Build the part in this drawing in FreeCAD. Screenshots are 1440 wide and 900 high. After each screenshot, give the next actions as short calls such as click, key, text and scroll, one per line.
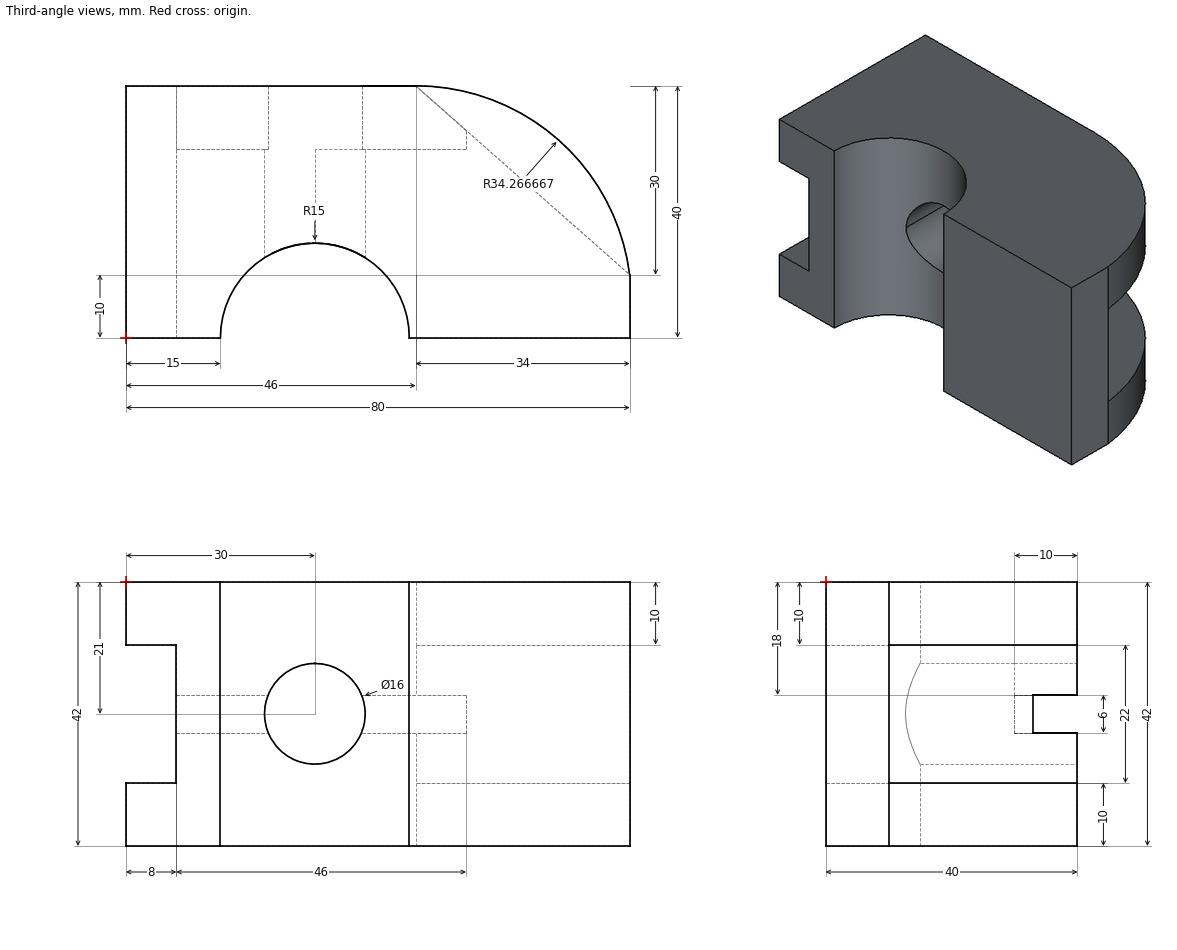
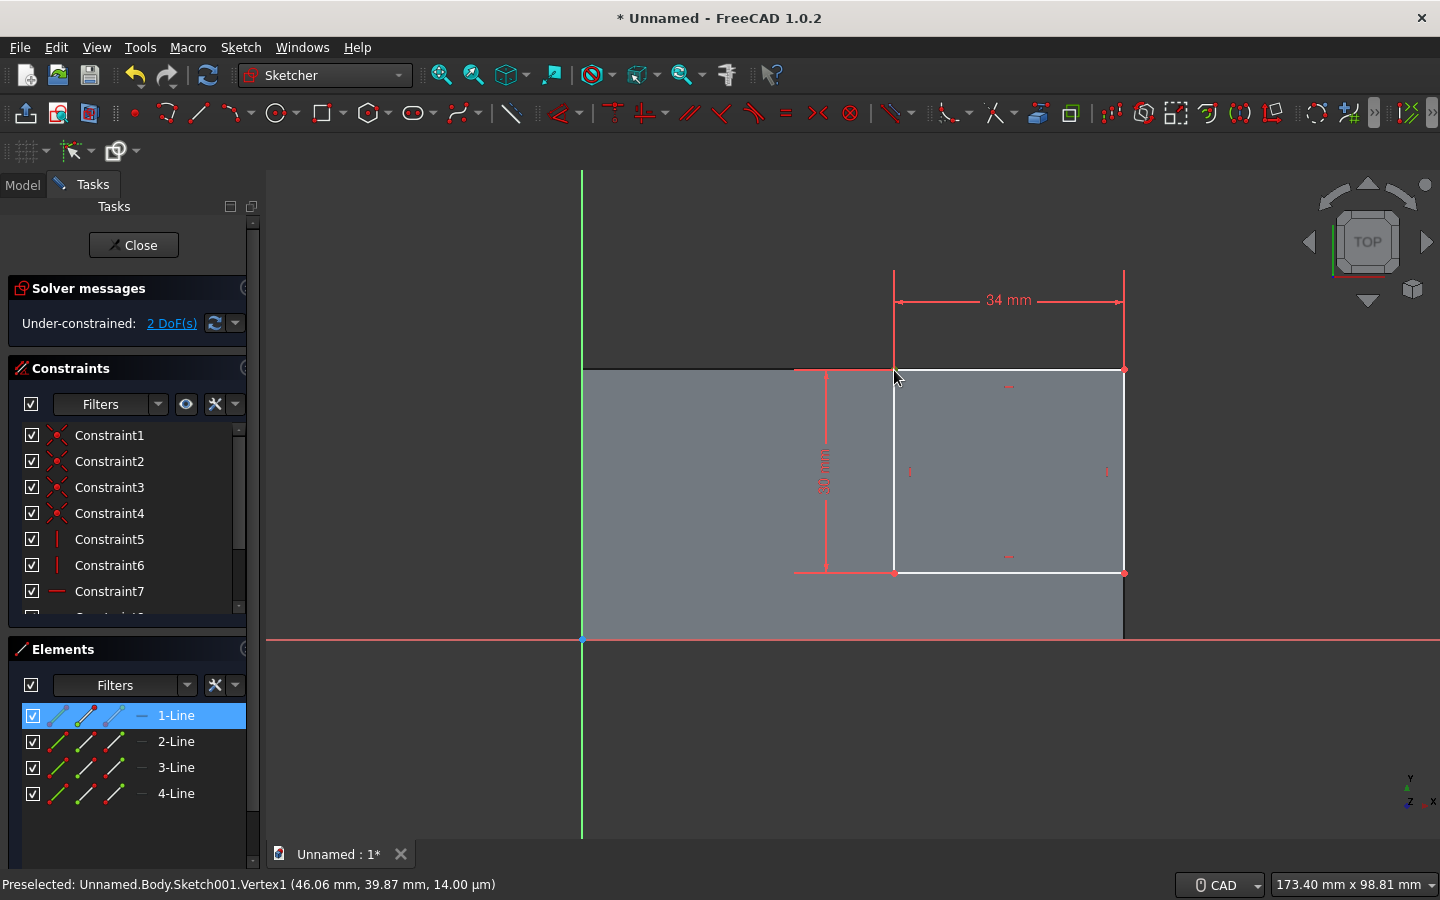
click(582, 114)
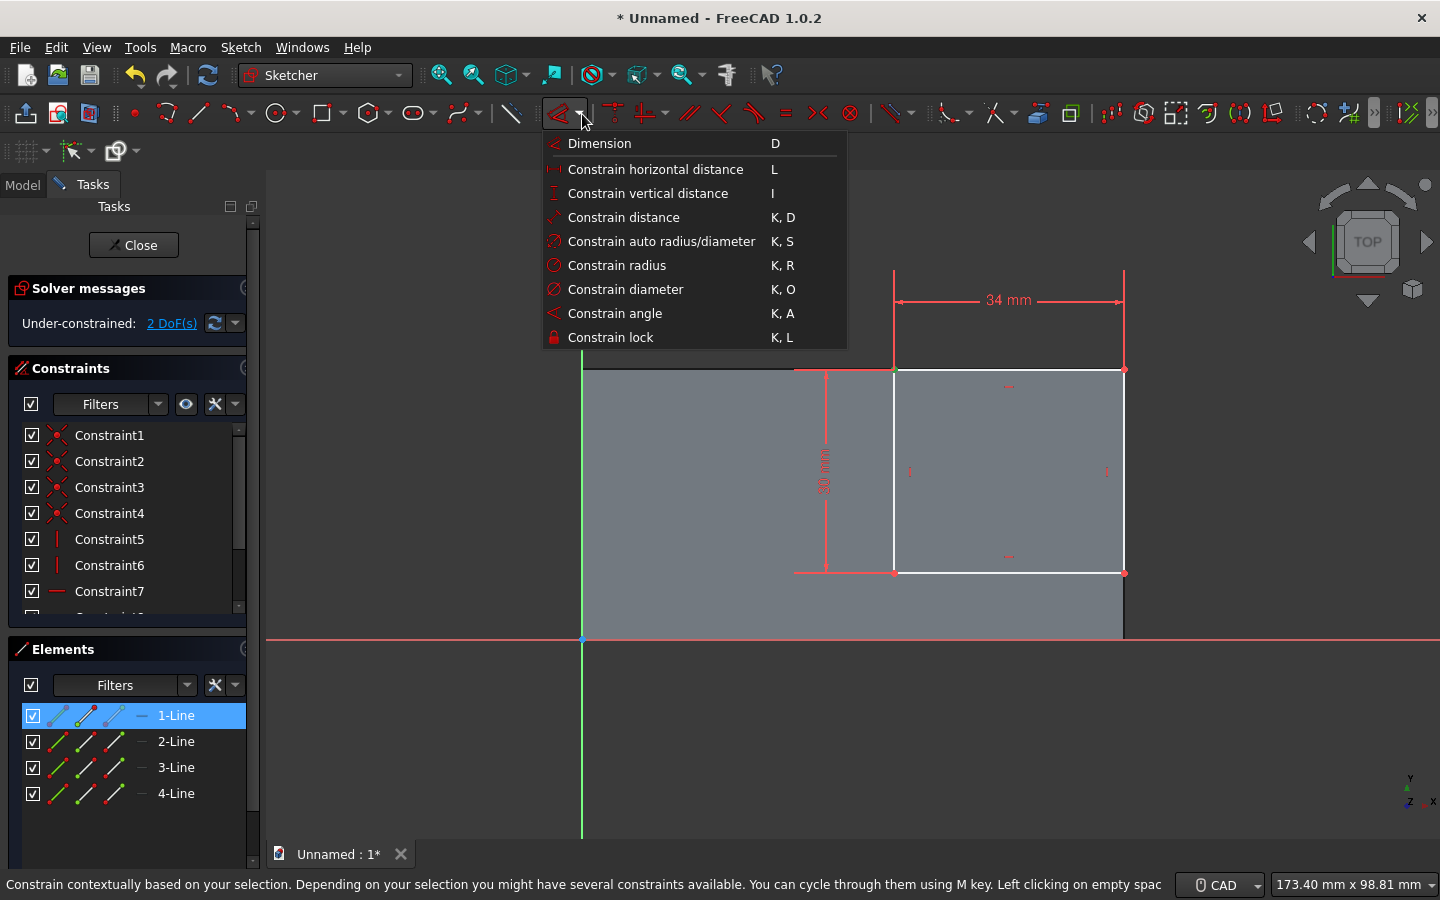
click(695, 169)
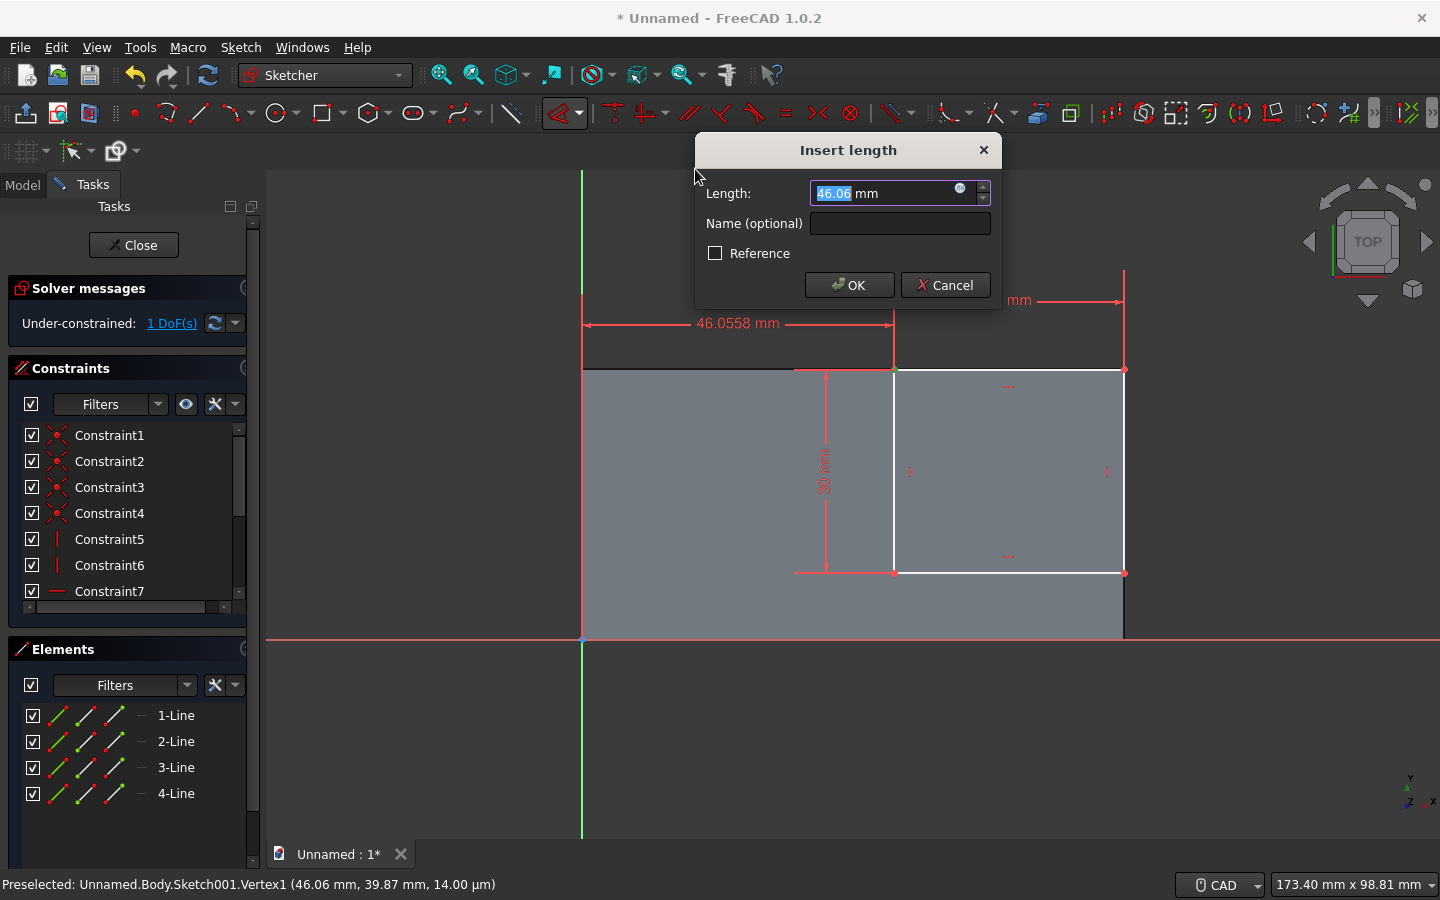
text(46)
key(Return)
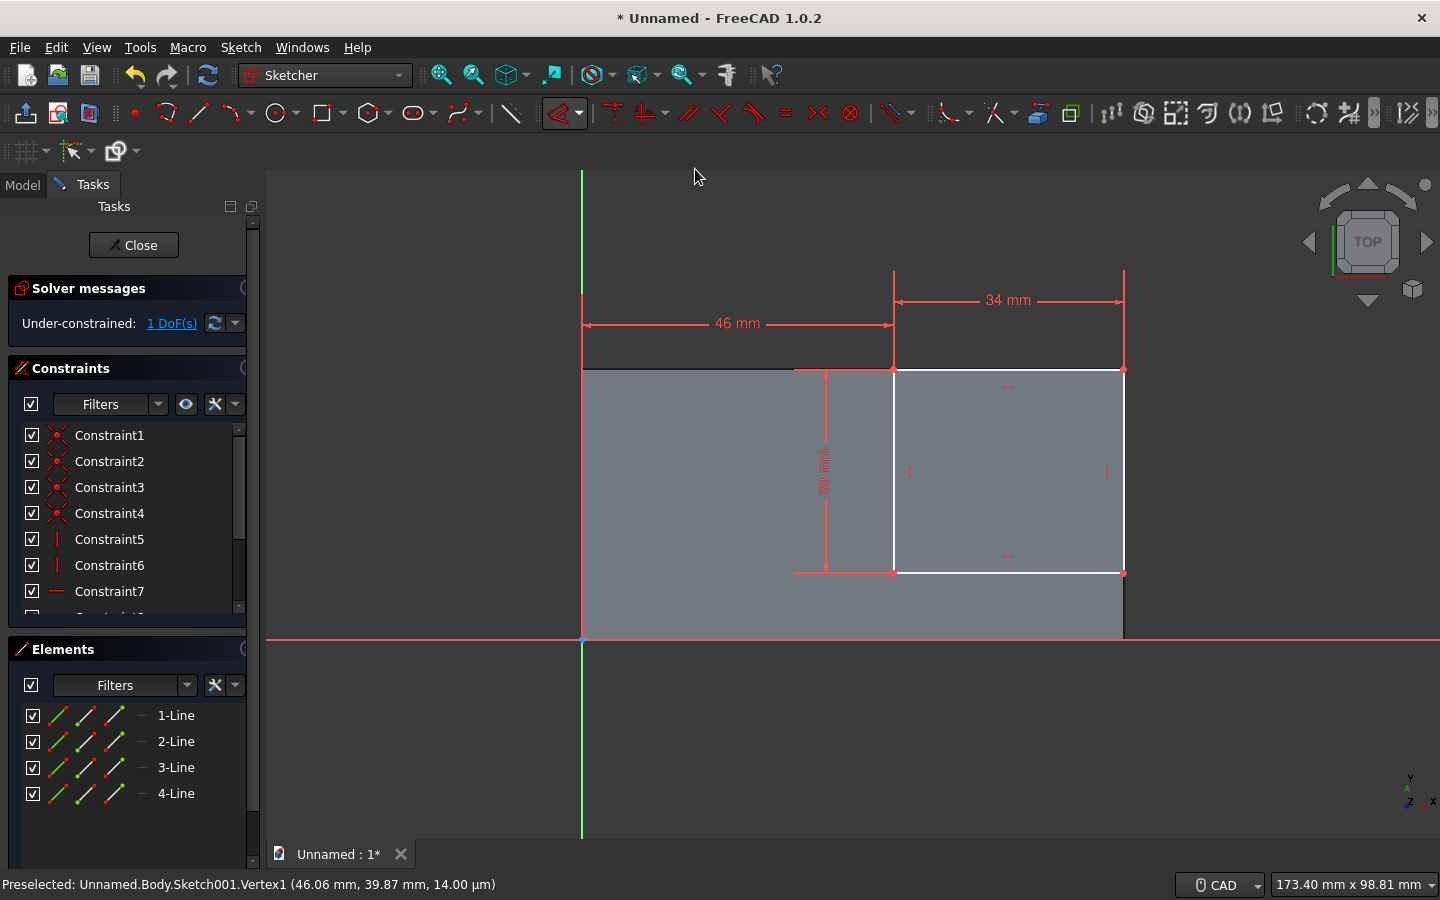
click(894, 370)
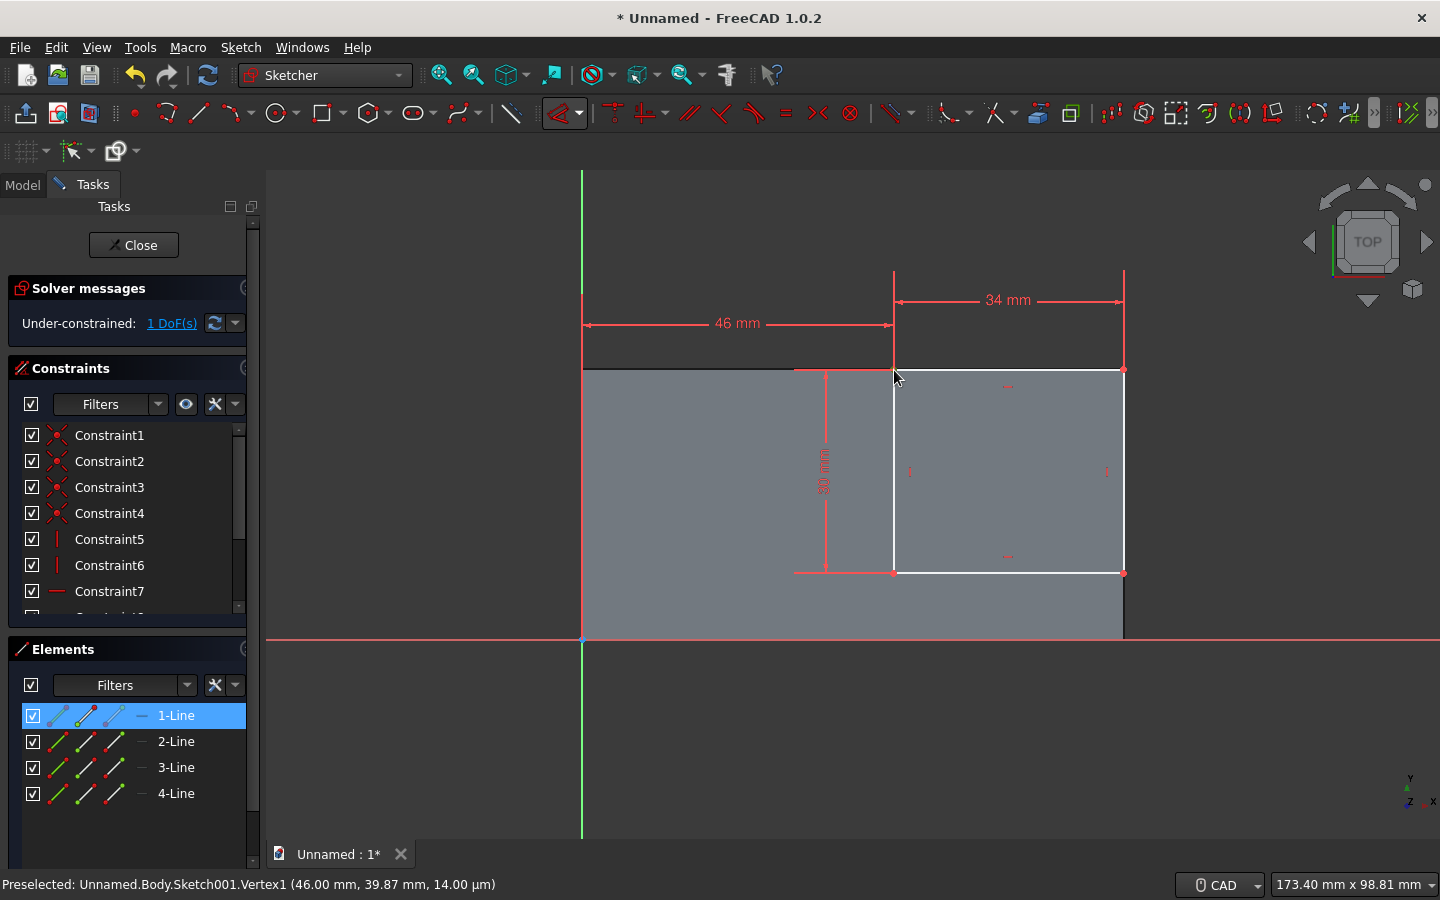
click(582, 114)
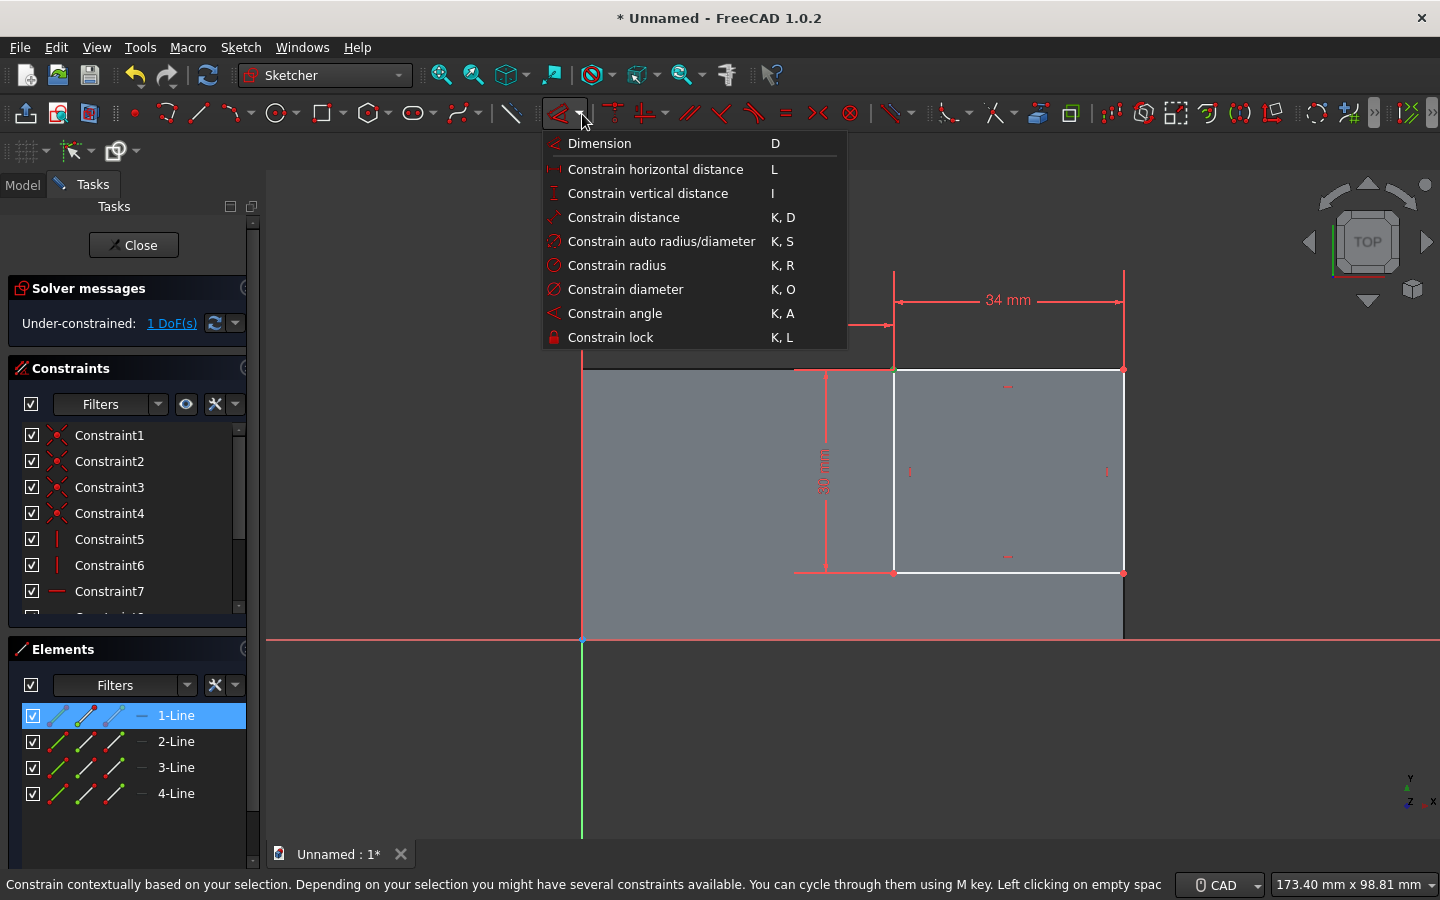
click(695, 193)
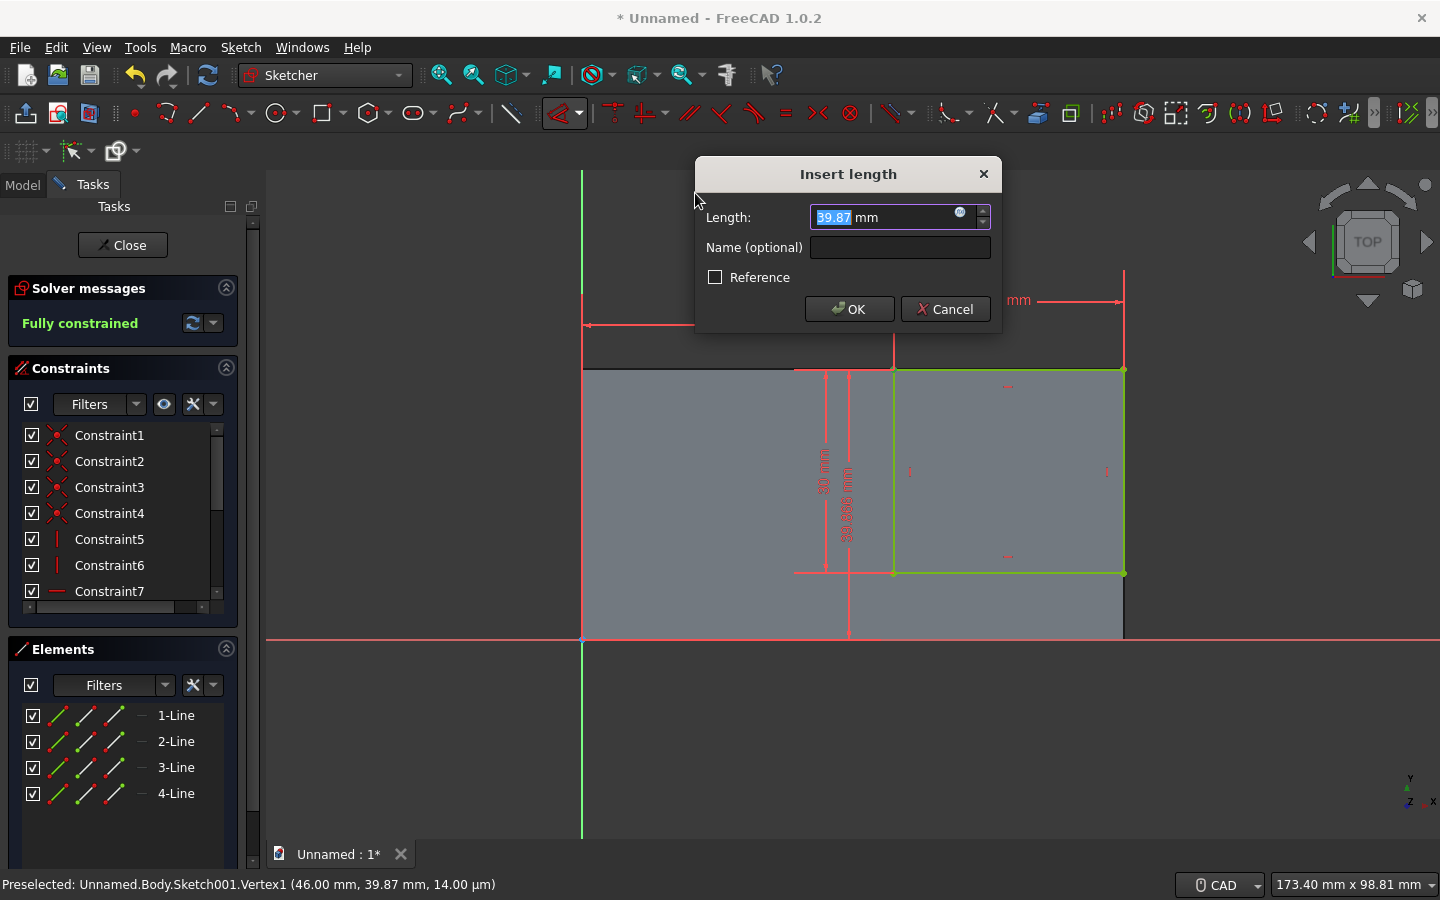
text(40)
key(Return)